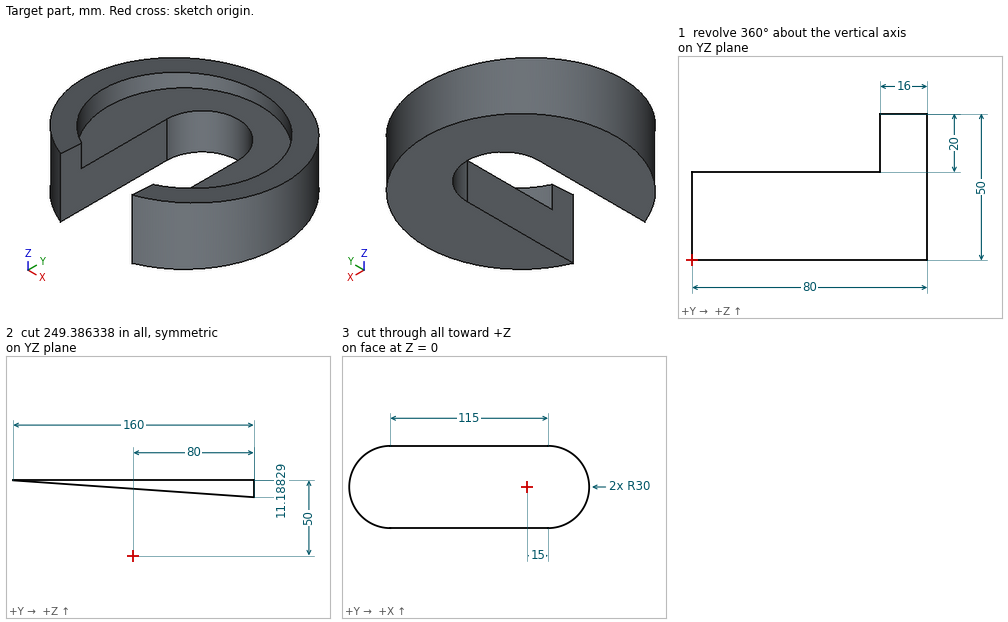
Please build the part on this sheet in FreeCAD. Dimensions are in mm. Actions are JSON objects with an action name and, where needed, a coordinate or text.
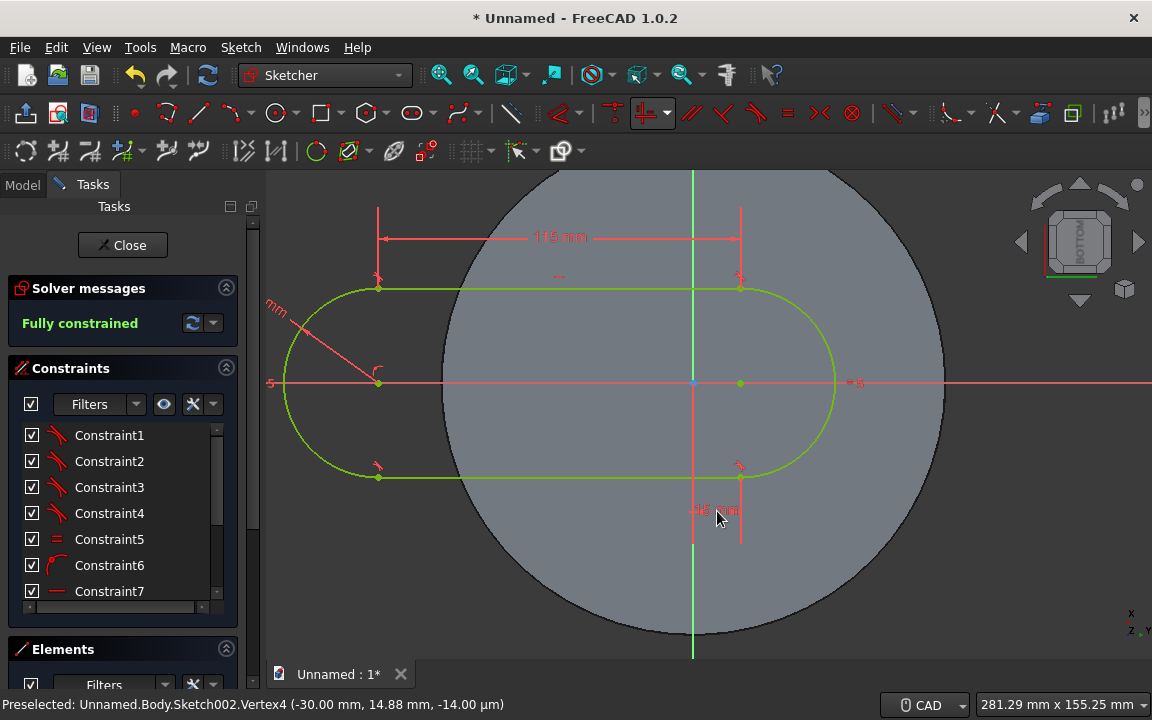
{"action": "left_click", "coordinate": [123, 245]}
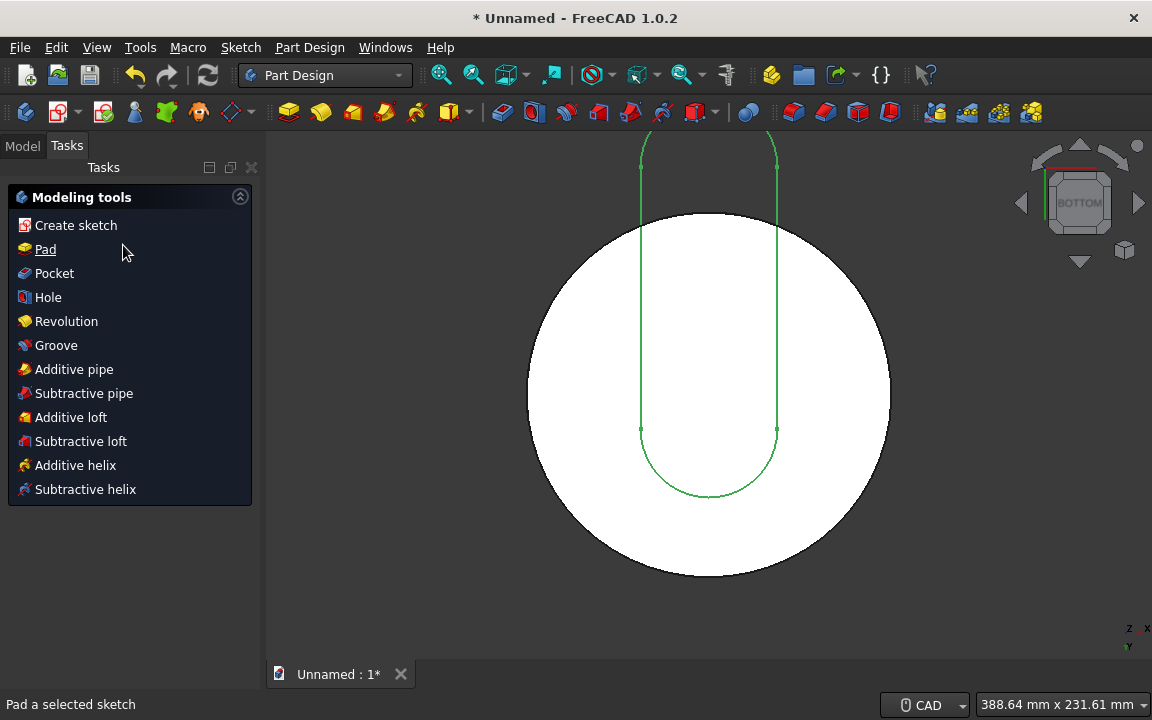
{"action": "left_click", "coordinate": [504, 112]}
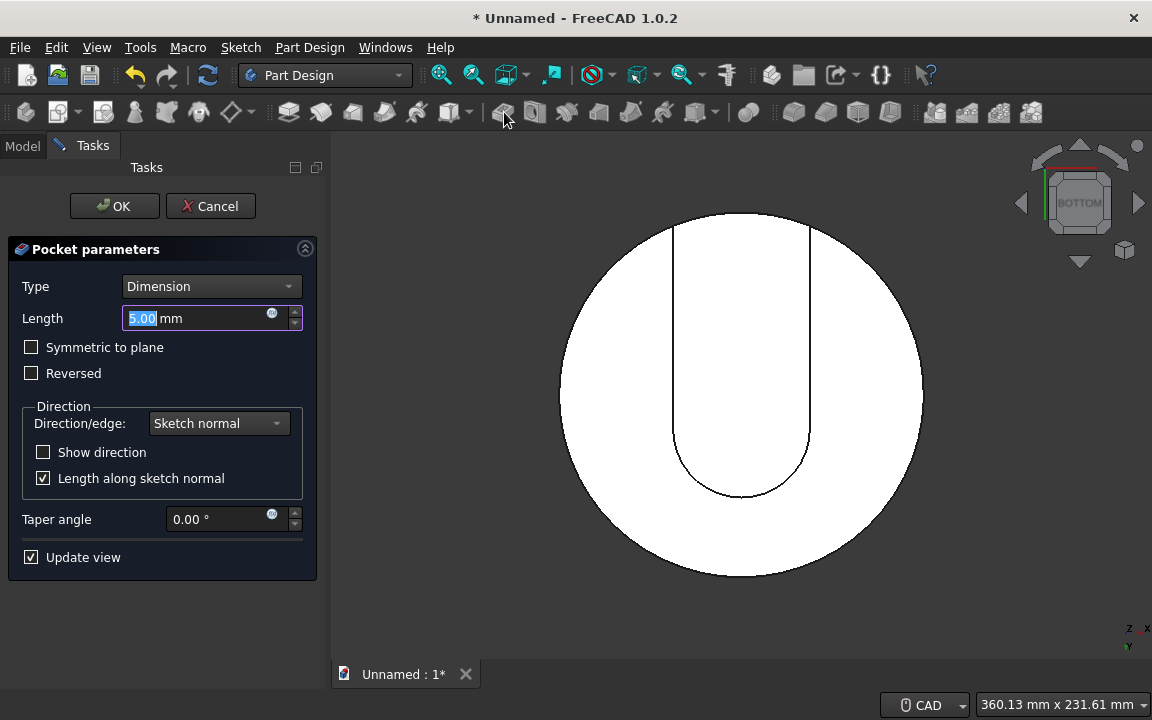
{"action": "left_click", "coordinate": [212, 286]}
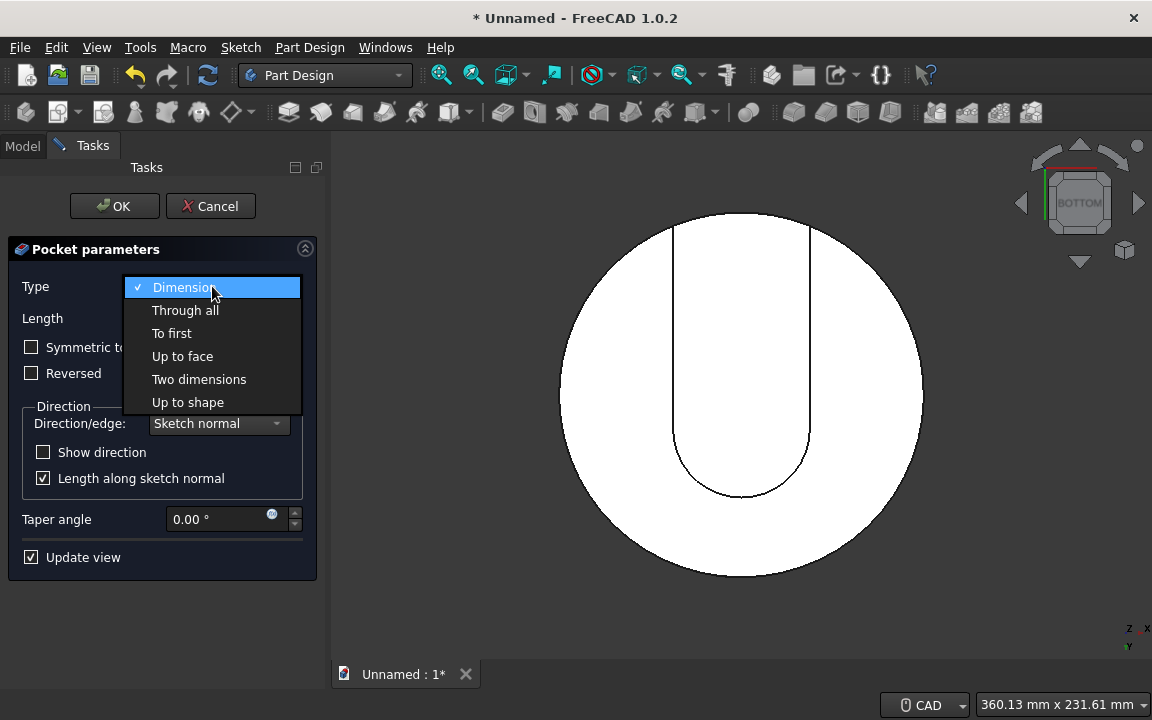
{"action": "left_click", "coordinate": [212, 310]}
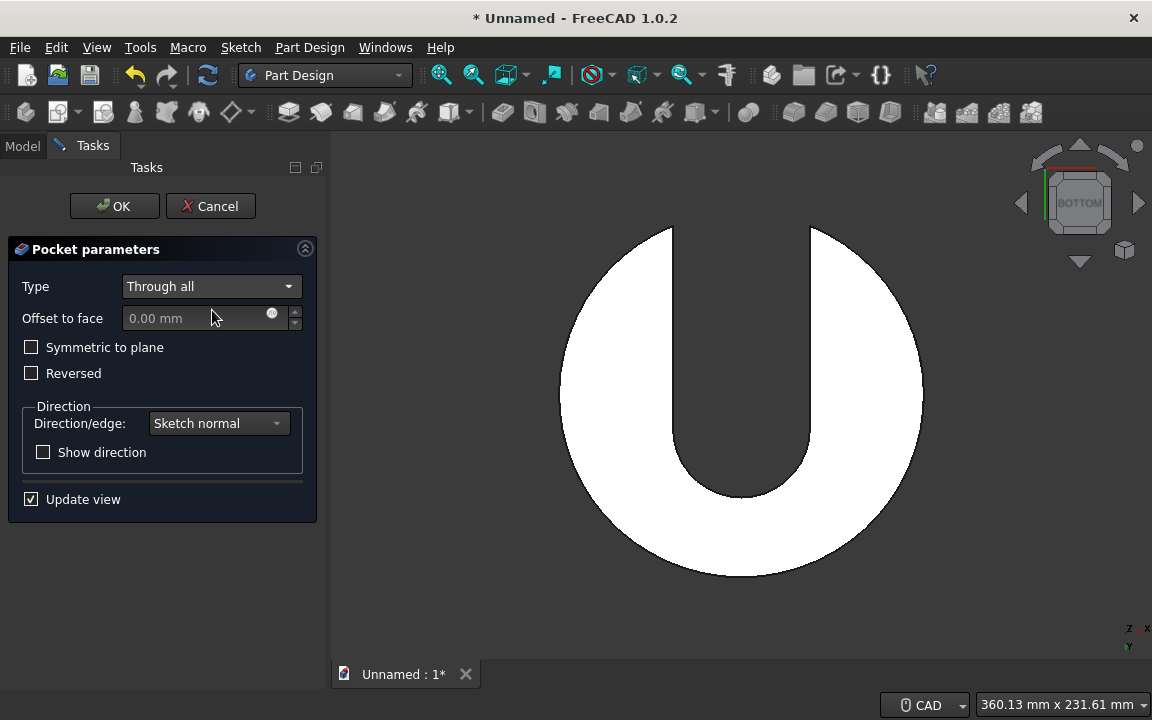
{"action": "left_click", "coordinate": [115, 206]}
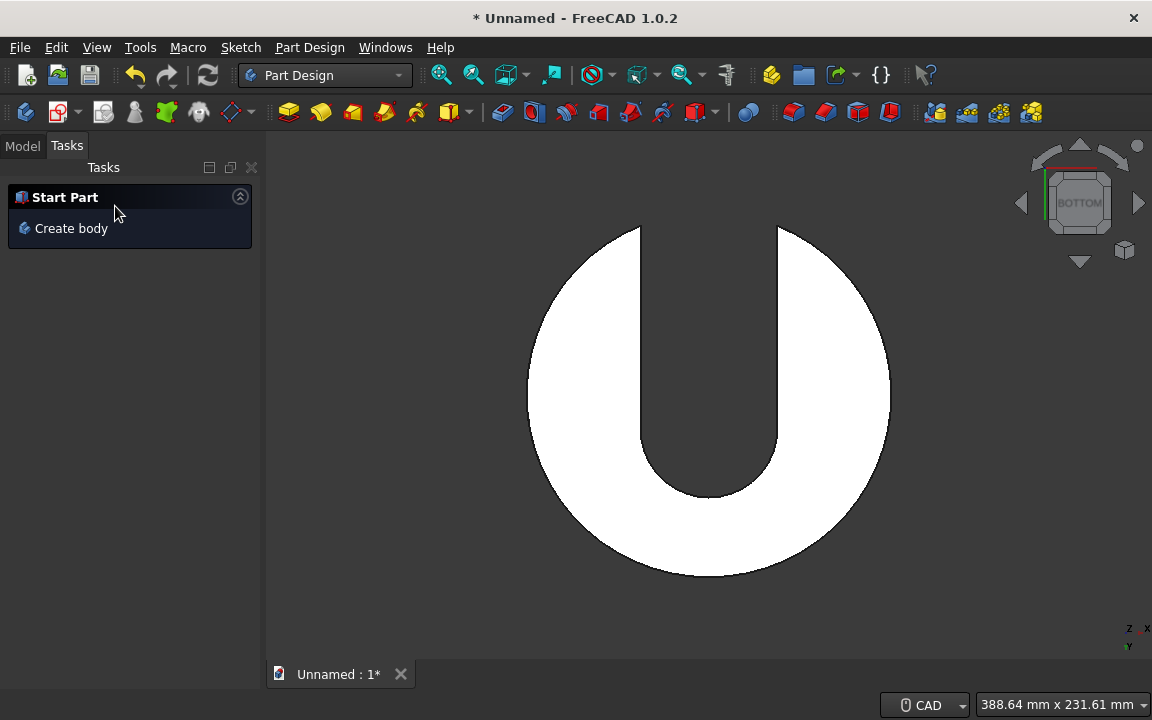
{"action": "key", "text": "0"}